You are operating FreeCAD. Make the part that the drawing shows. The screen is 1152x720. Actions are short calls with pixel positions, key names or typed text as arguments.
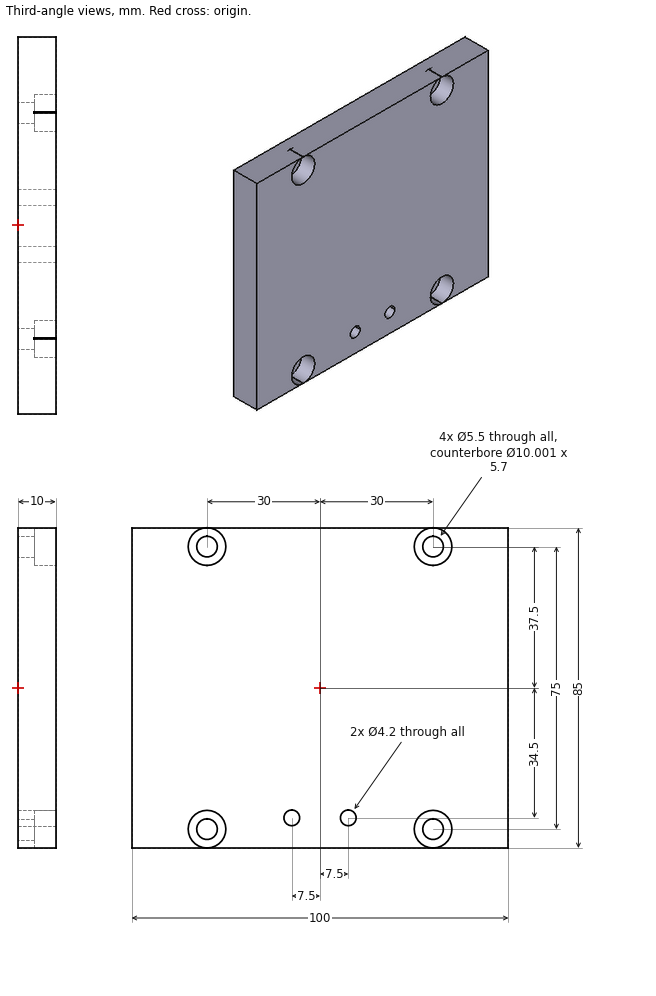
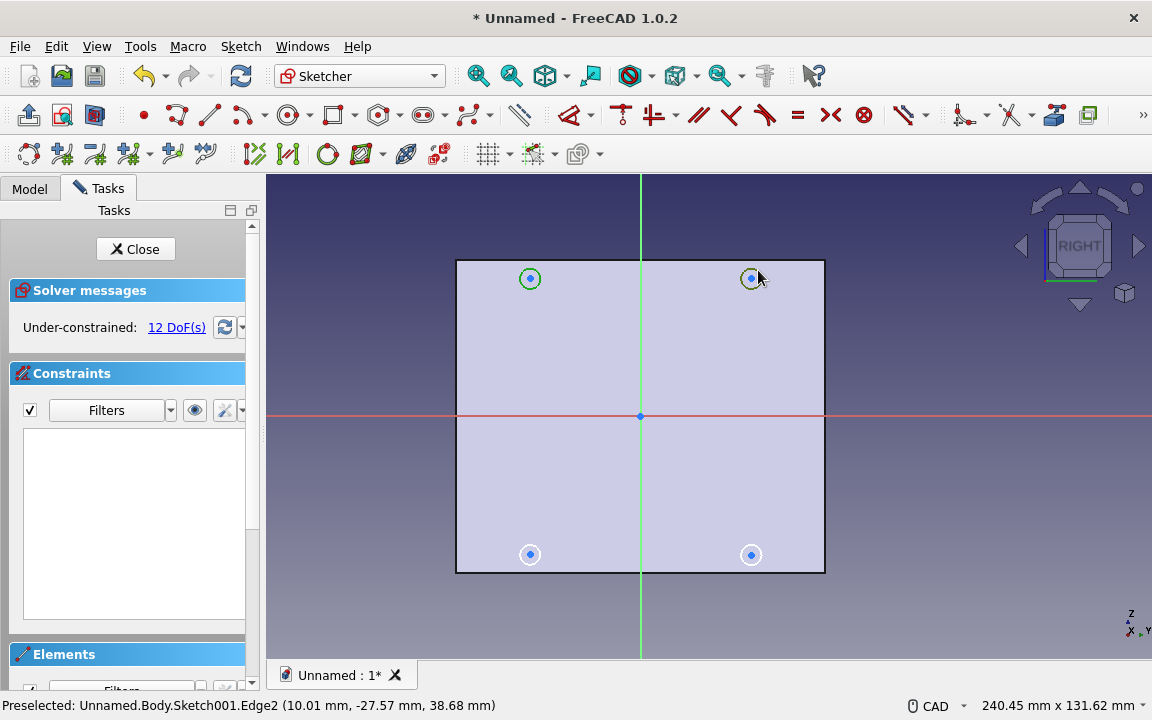
scroll(759, 548, up, 2)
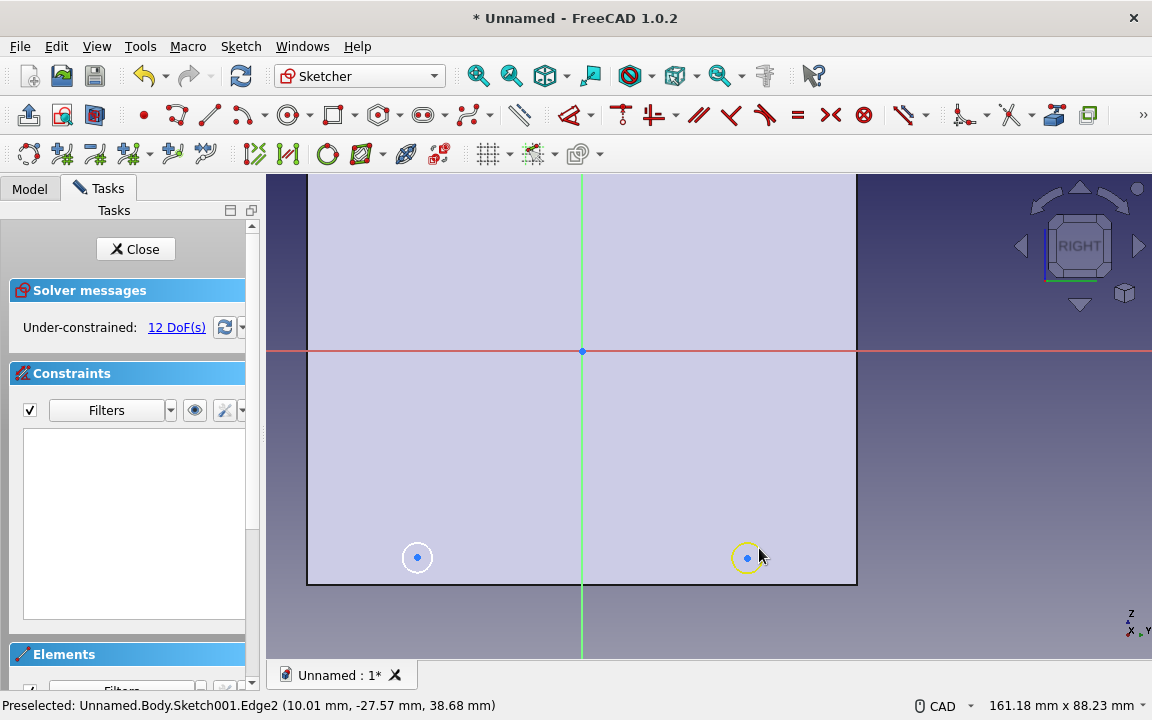
click(758, 547)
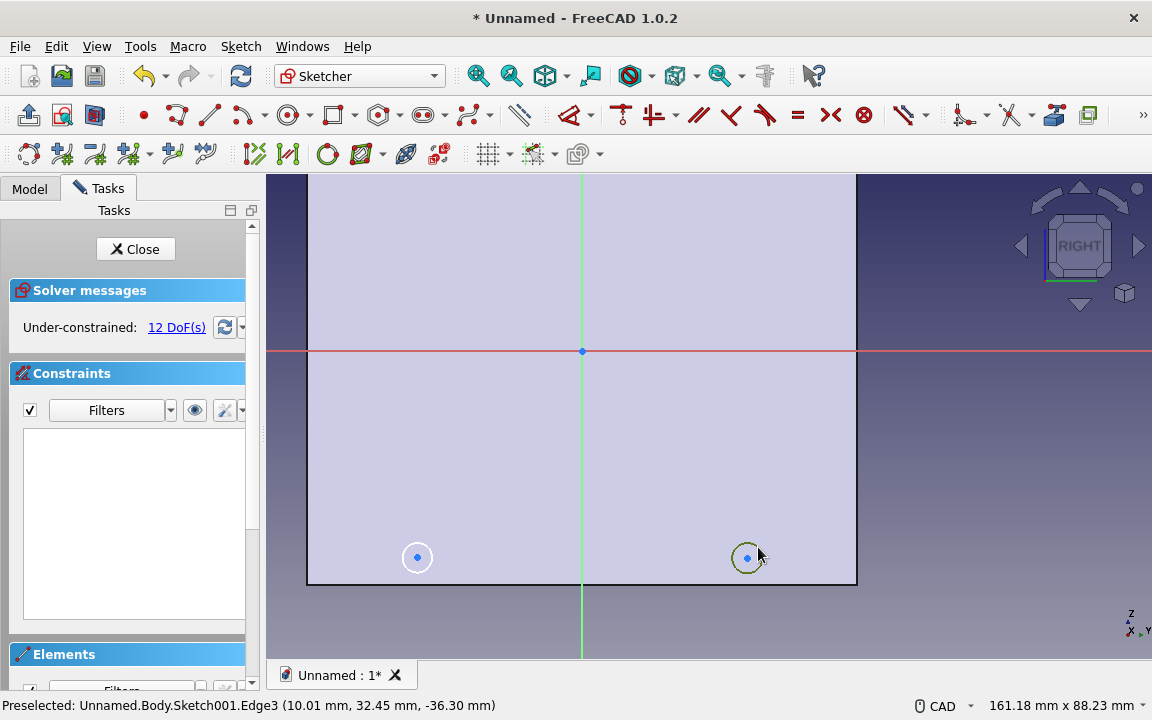
click(428, 547)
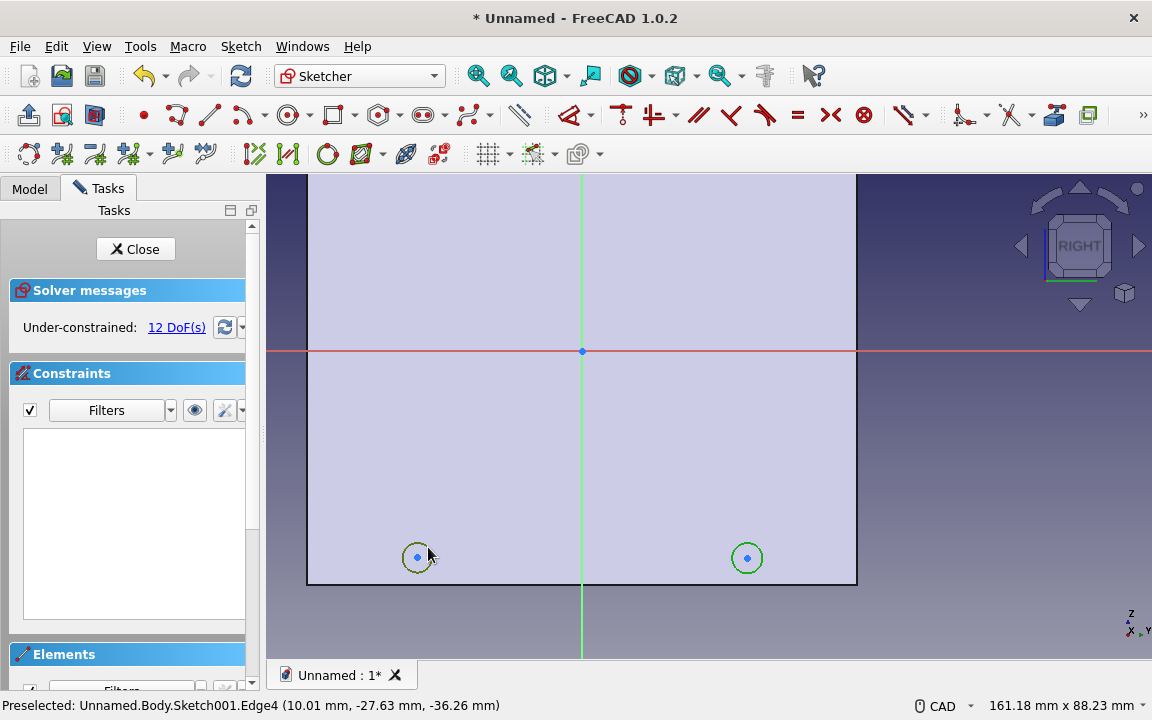
click(798, 116)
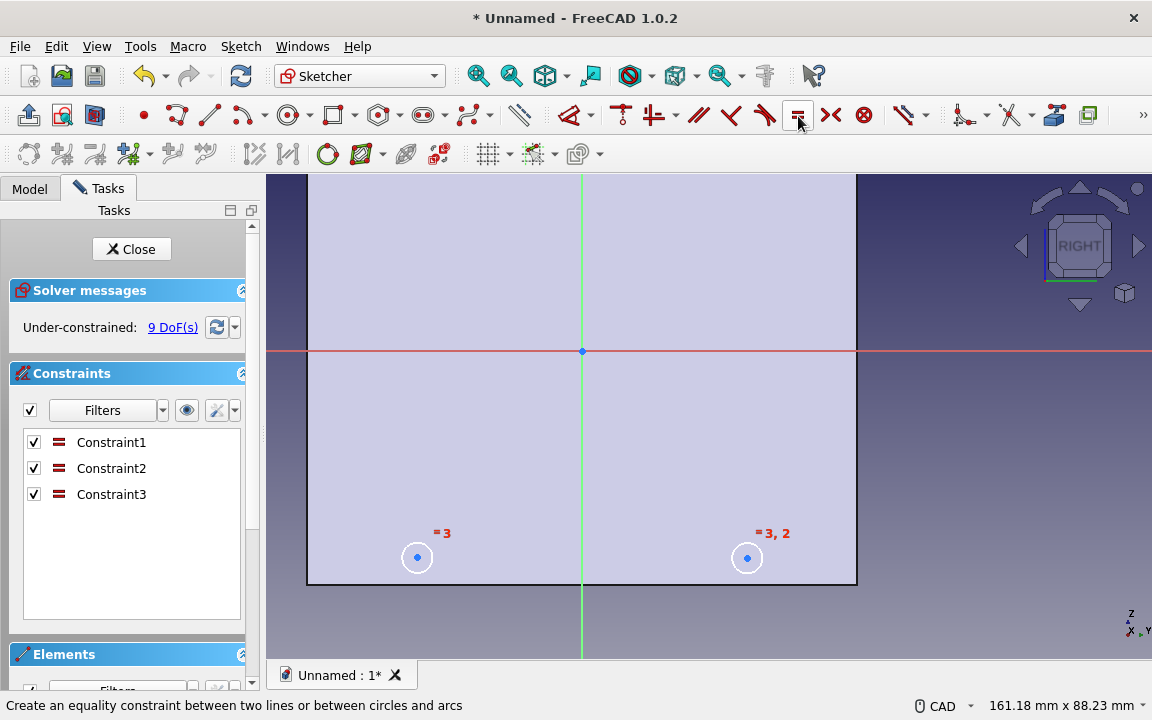
scroll(759, 549, down, 2)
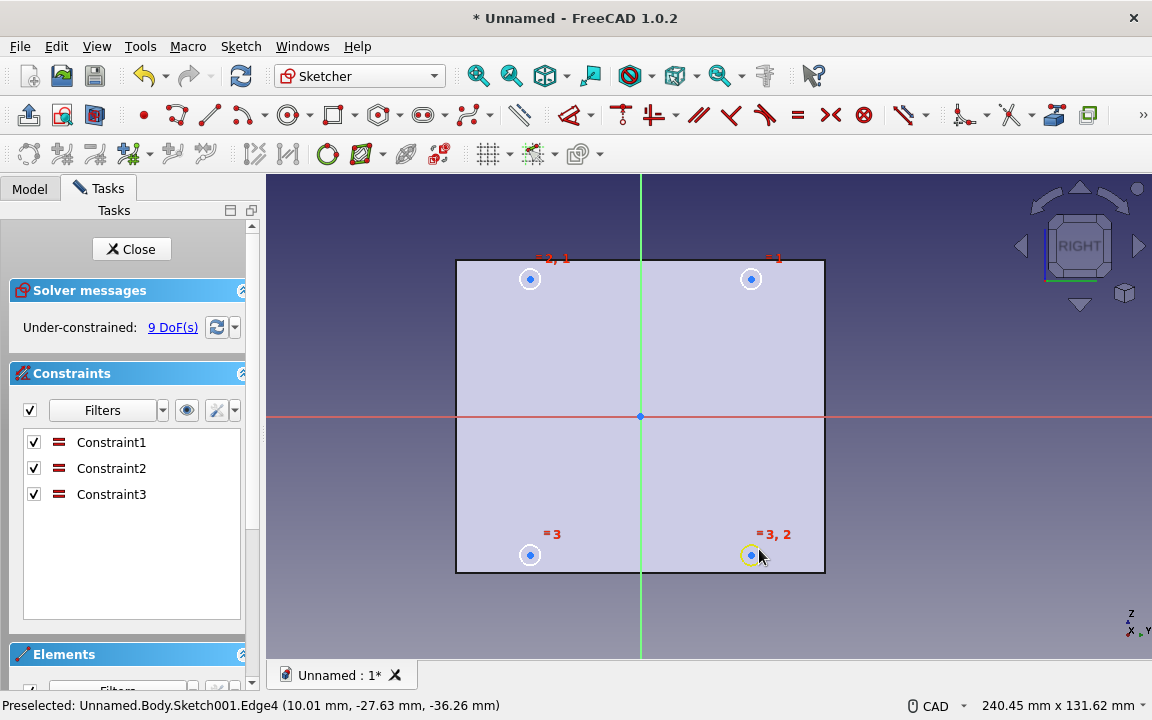
click(751, 279)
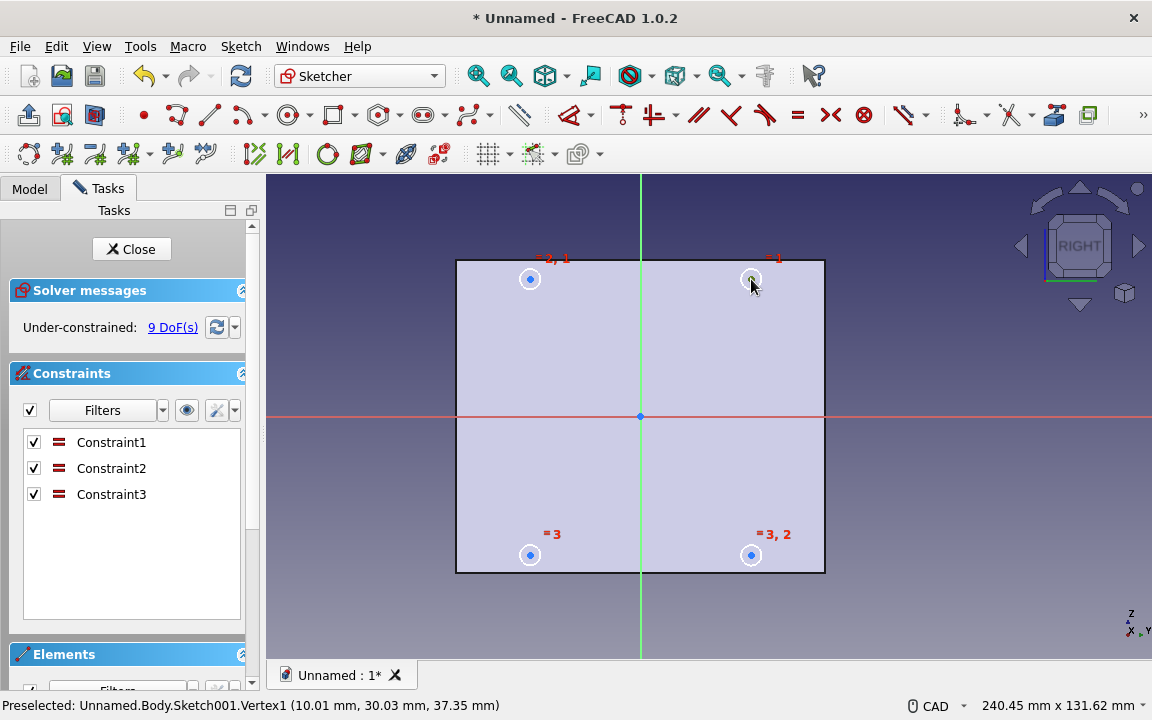
click(530, 279)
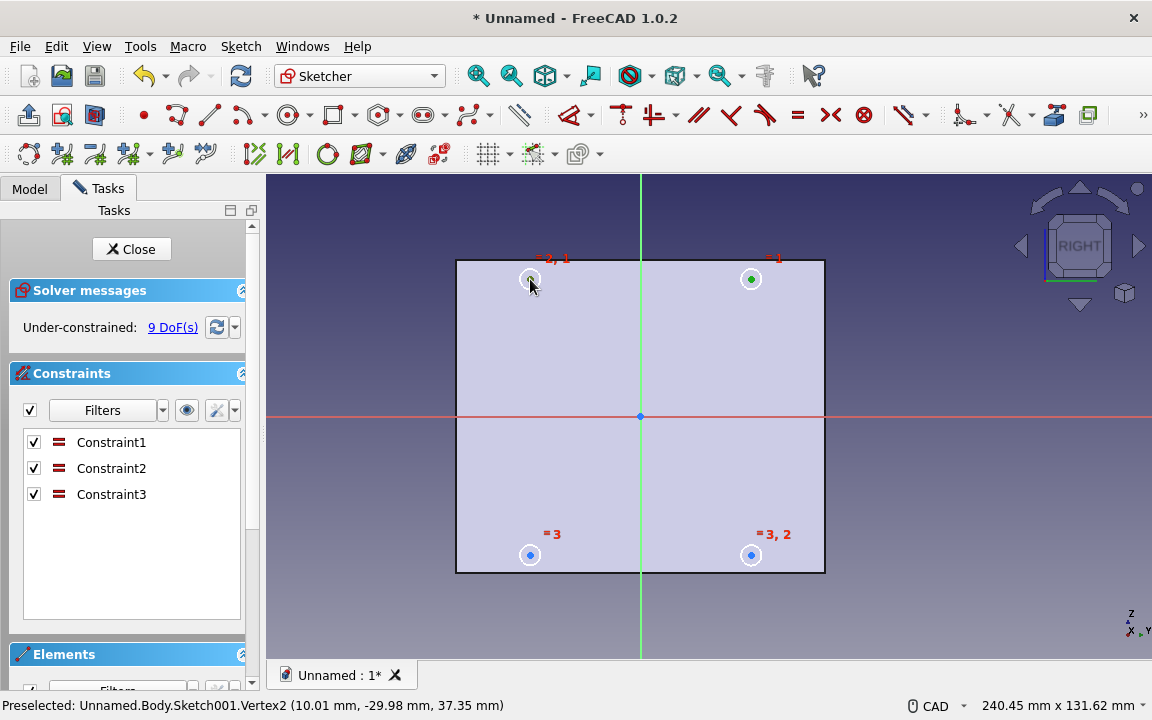
click(676, 116)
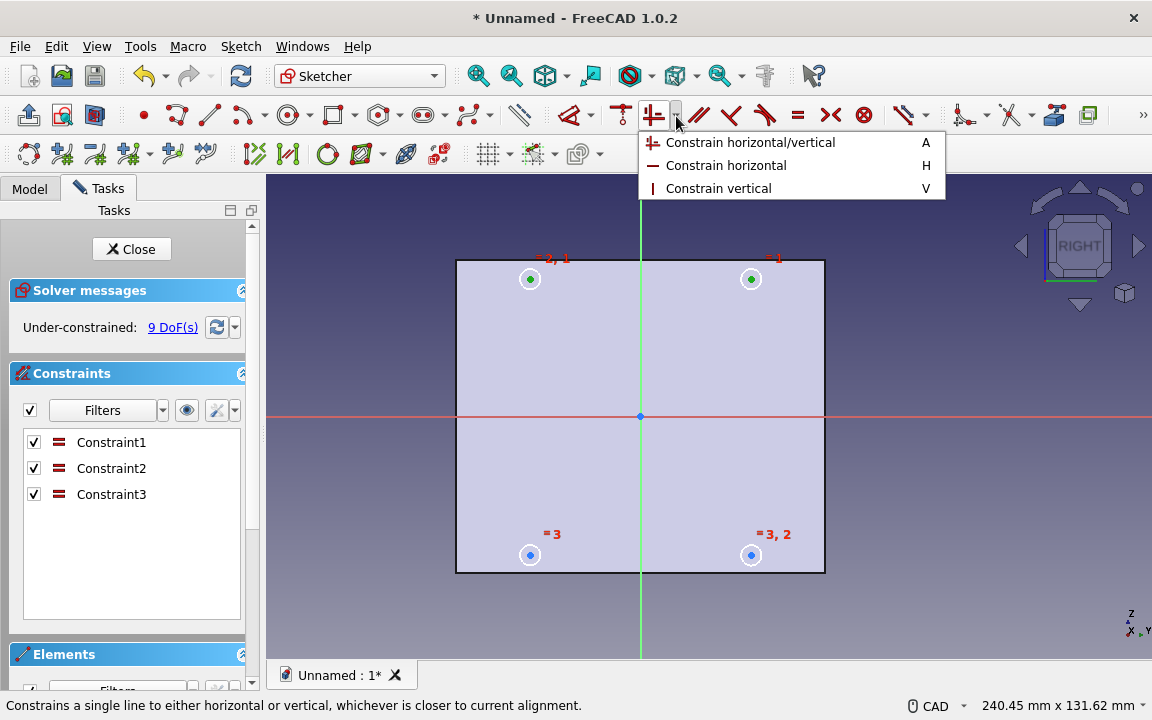
click(792, 166)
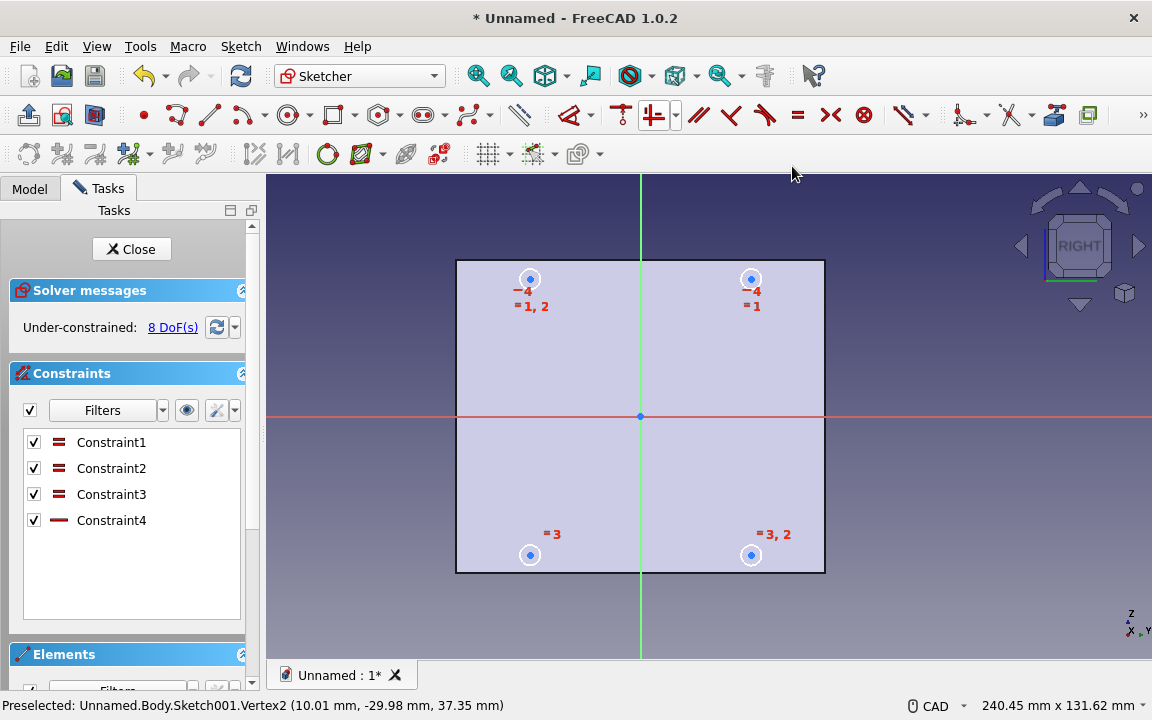
click(751, 279)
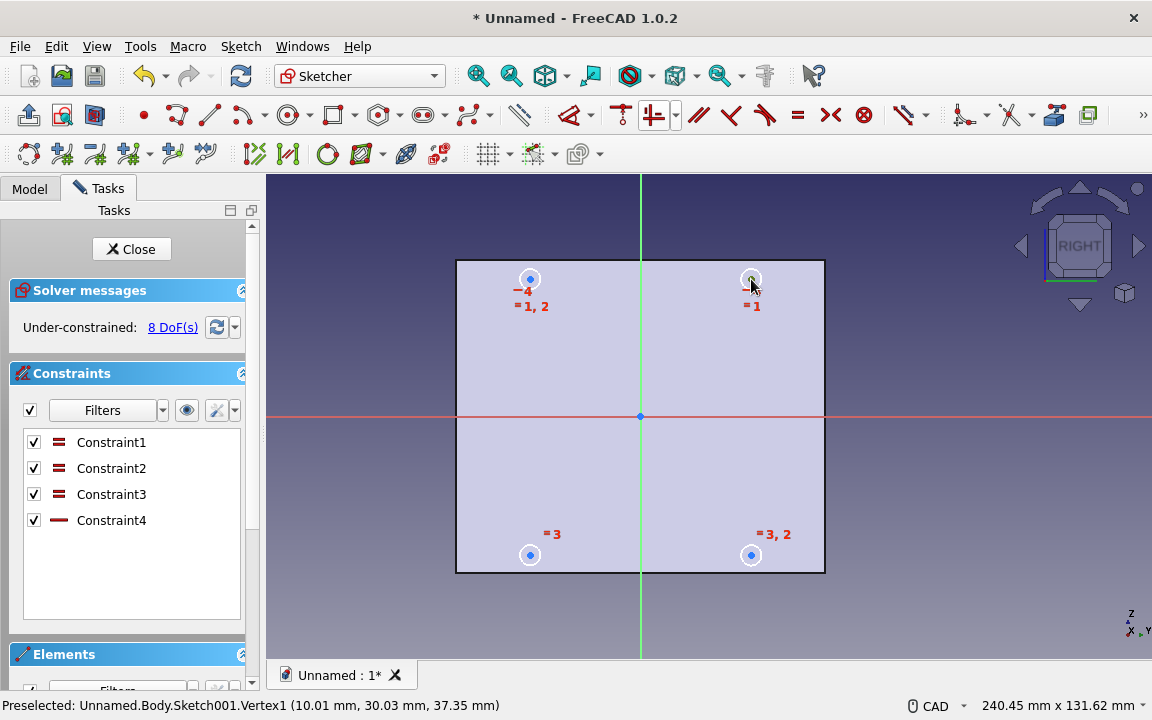
click(751, 555)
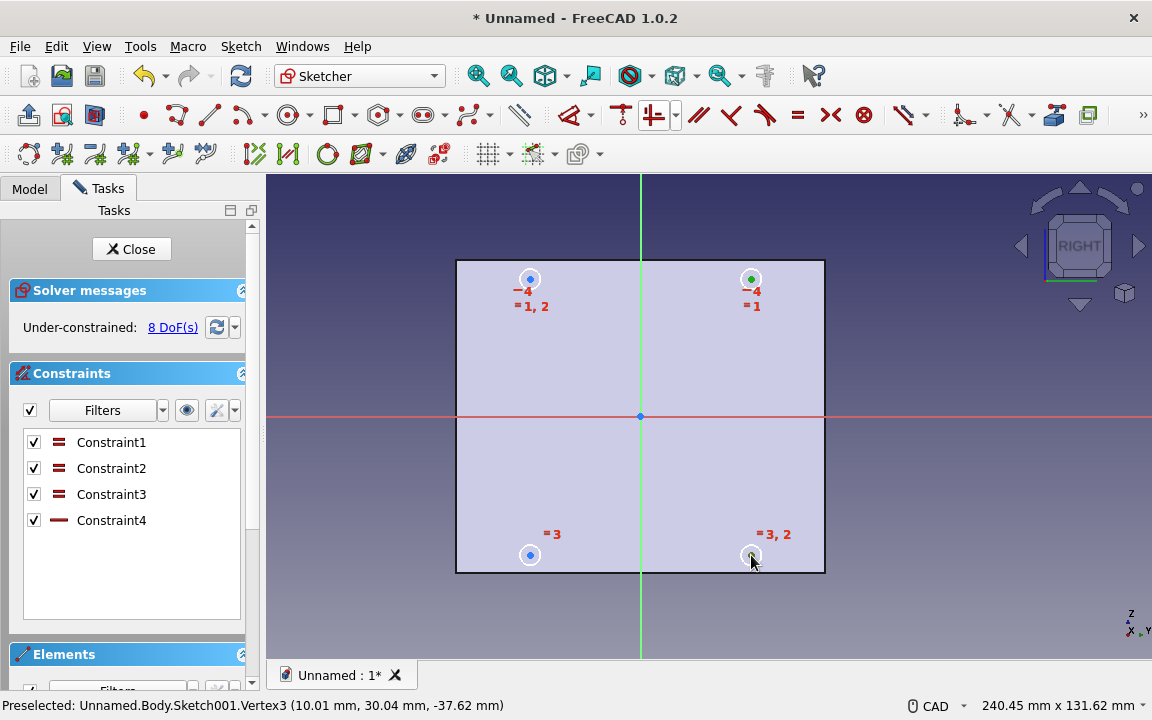
click(676, 116)